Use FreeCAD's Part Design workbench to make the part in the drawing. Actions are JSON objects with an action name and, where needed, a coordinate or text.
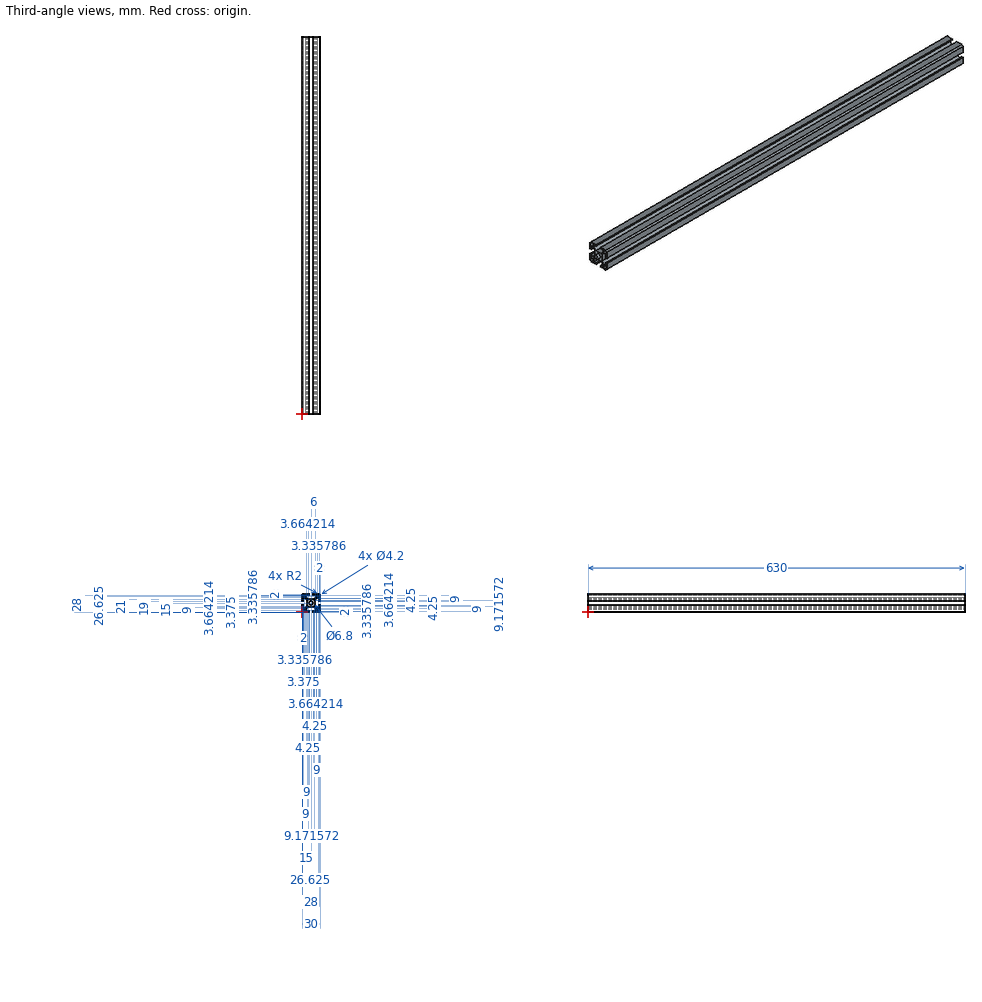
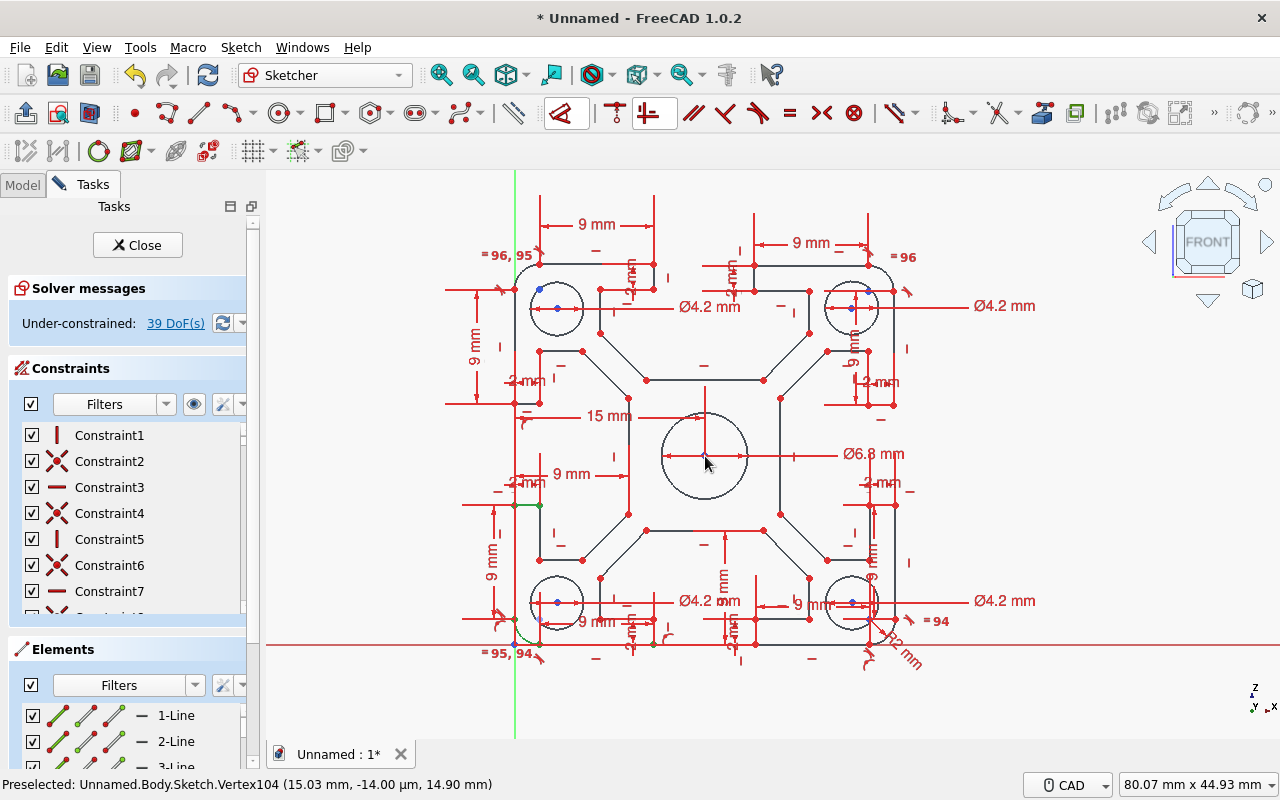
{"action": "left_click", "coordinate": [705, 456]}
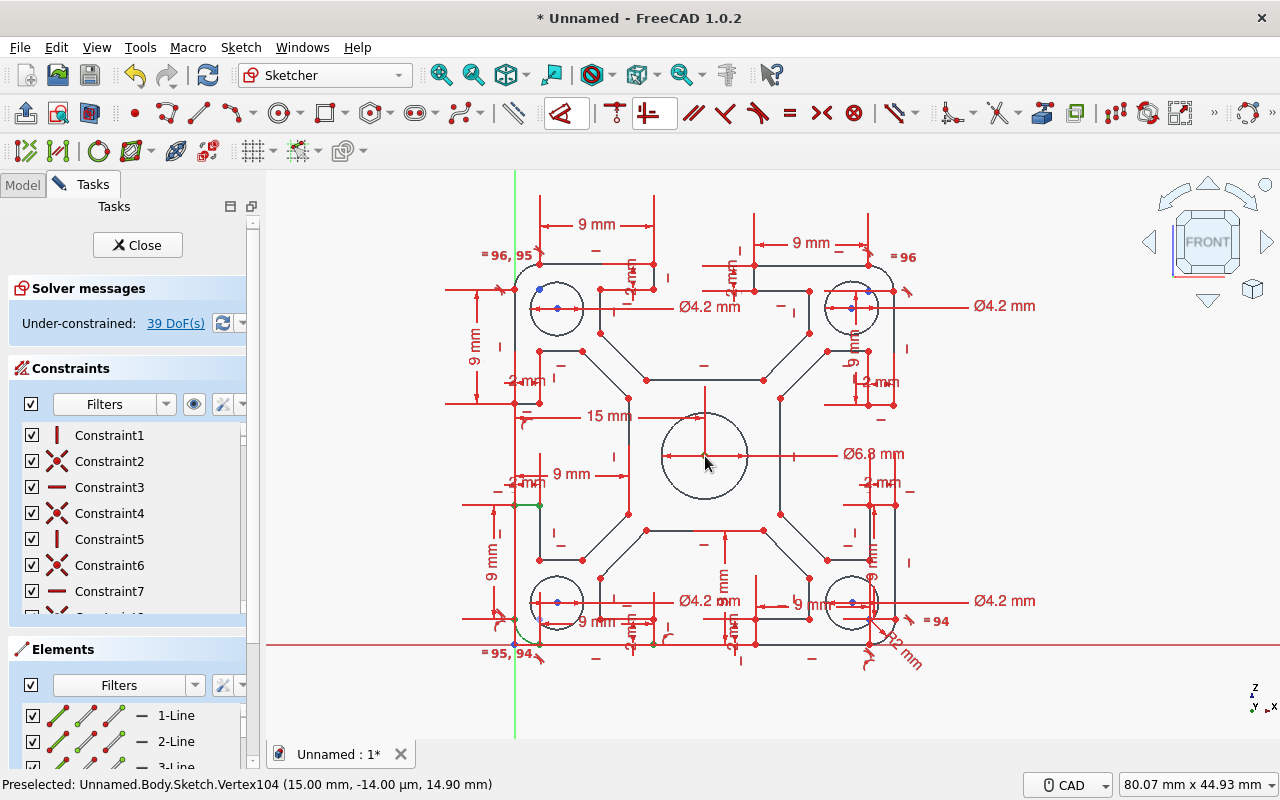
{"action": "left_click", "coordinate": [584, 114]}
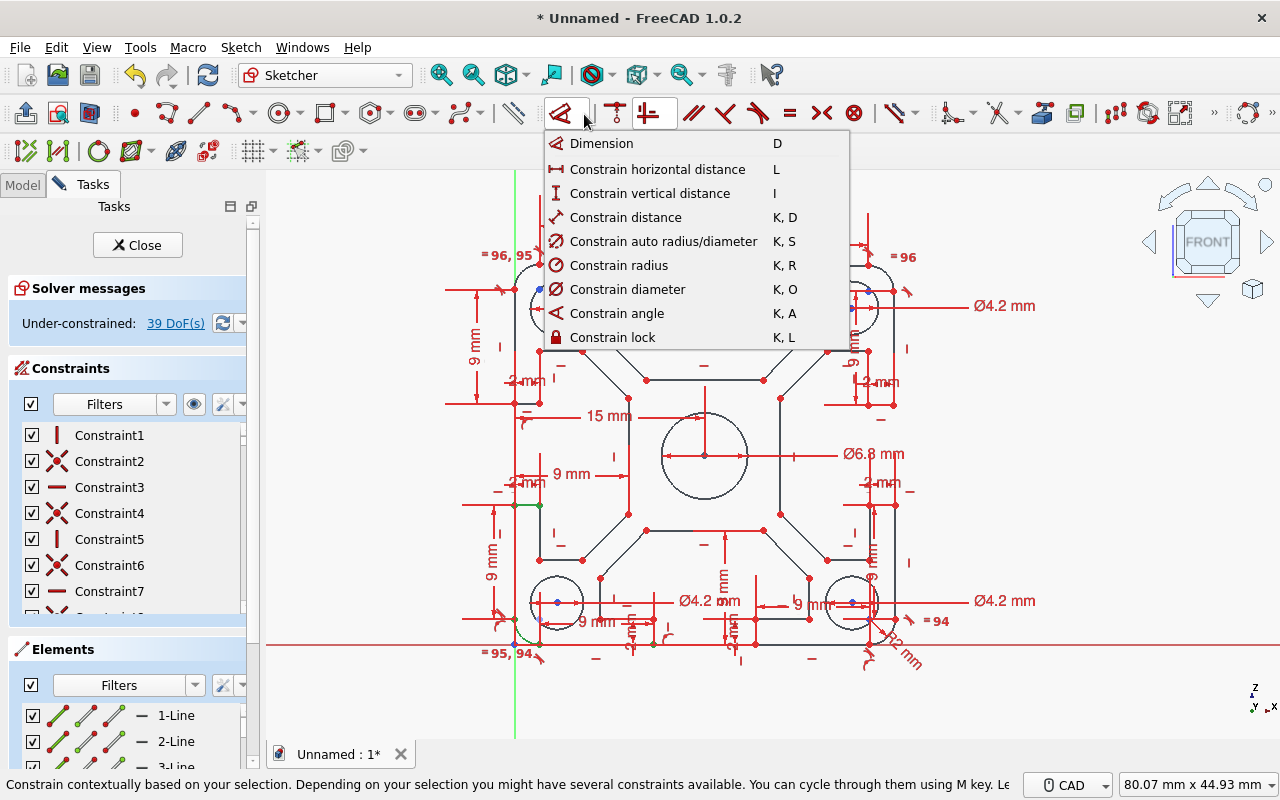
{"action": "left_click", "coordinate": [697, 193]}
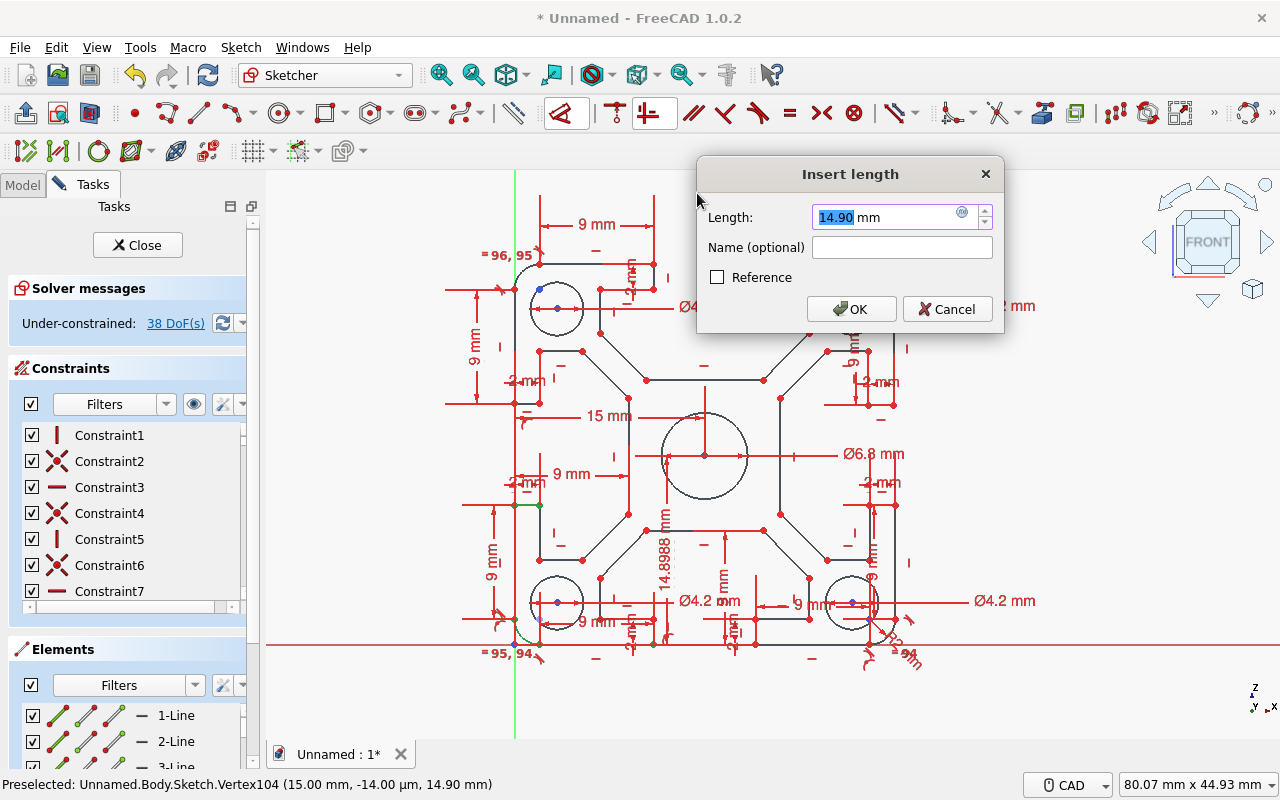
{"action": "type", "text": "15"}
{"action": "key", "text": "Return"}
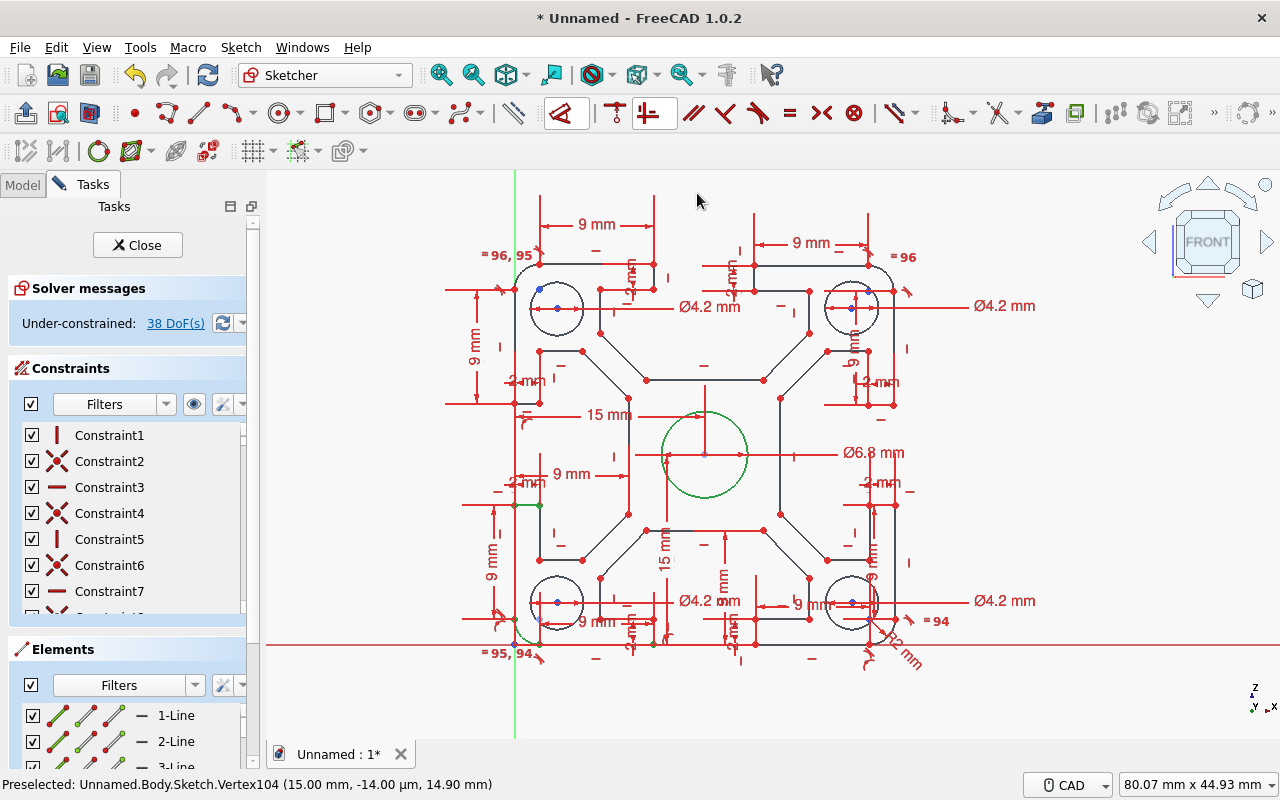
{"action": "left_click", "coordinate": [780, 398]}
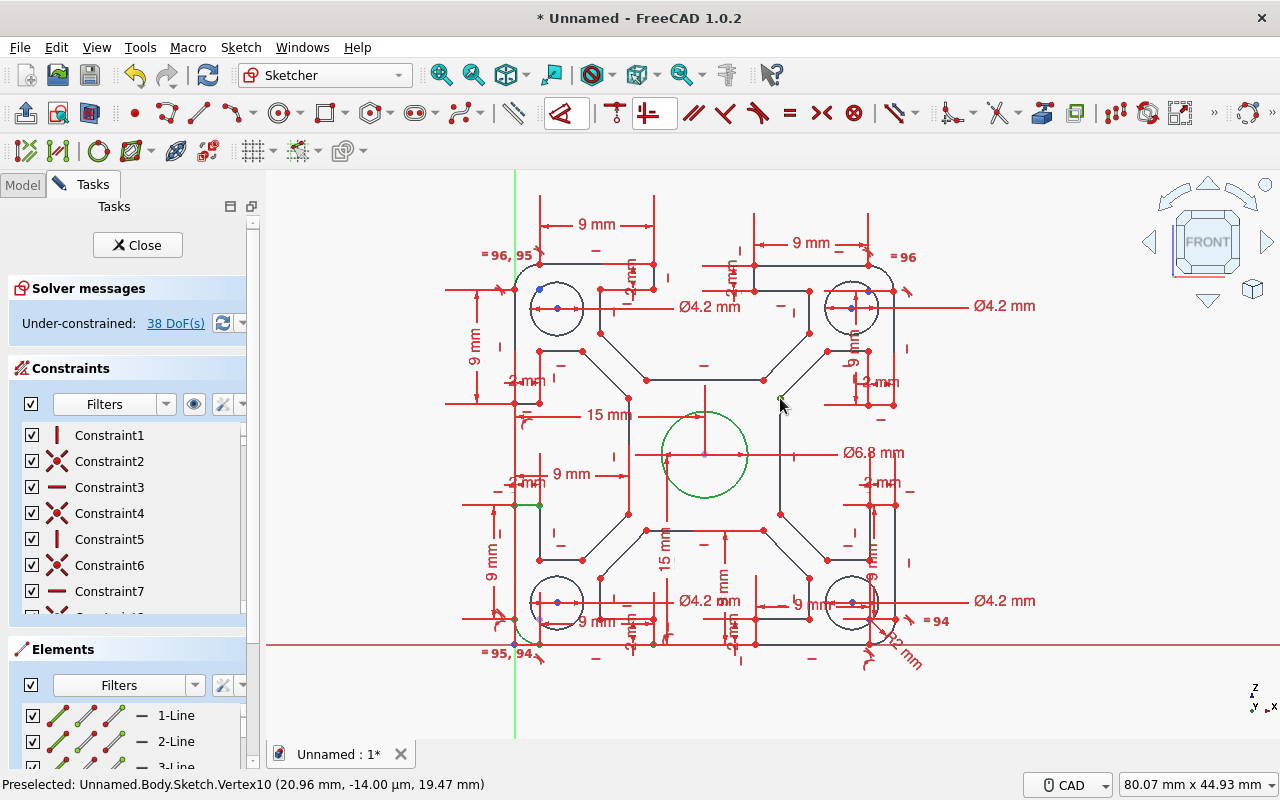
{"action": "left_click", "coordinate": [705, 455]}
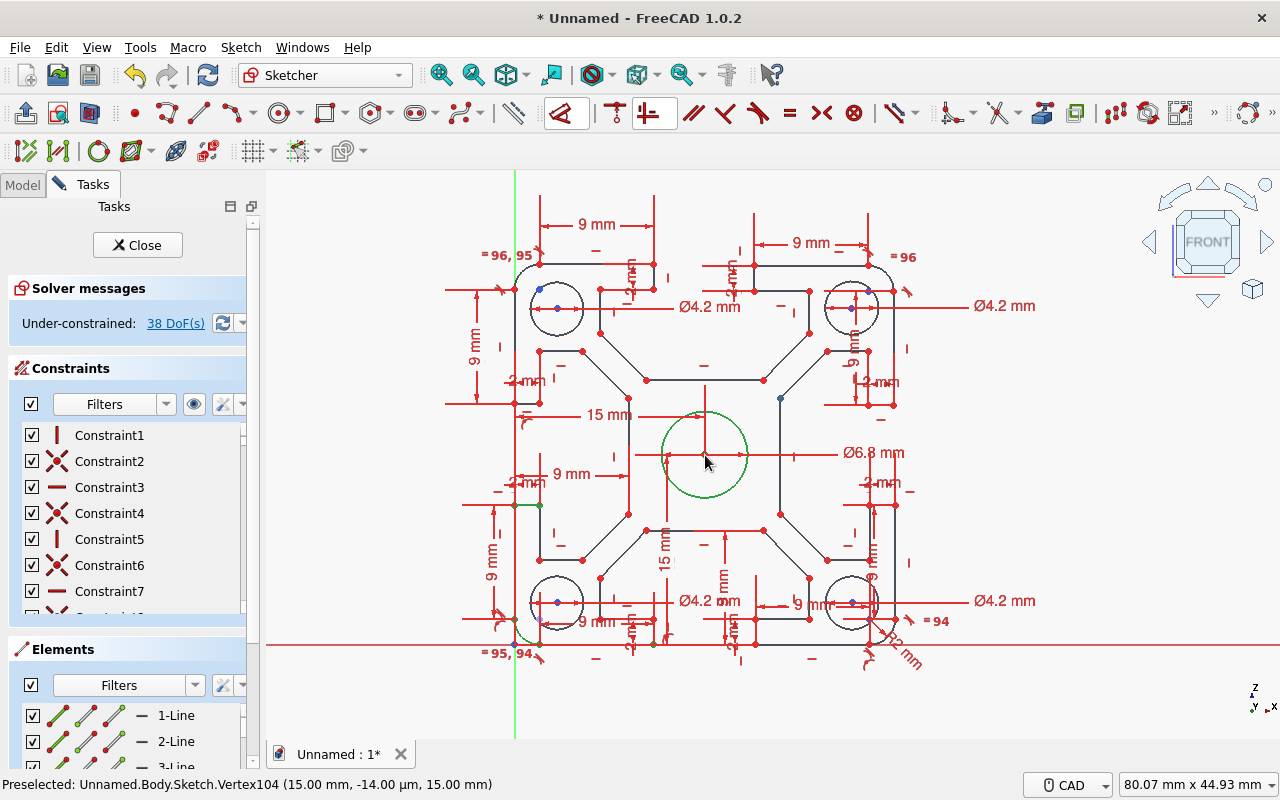
{"action": "left_click", "coordinate": [584, 114]}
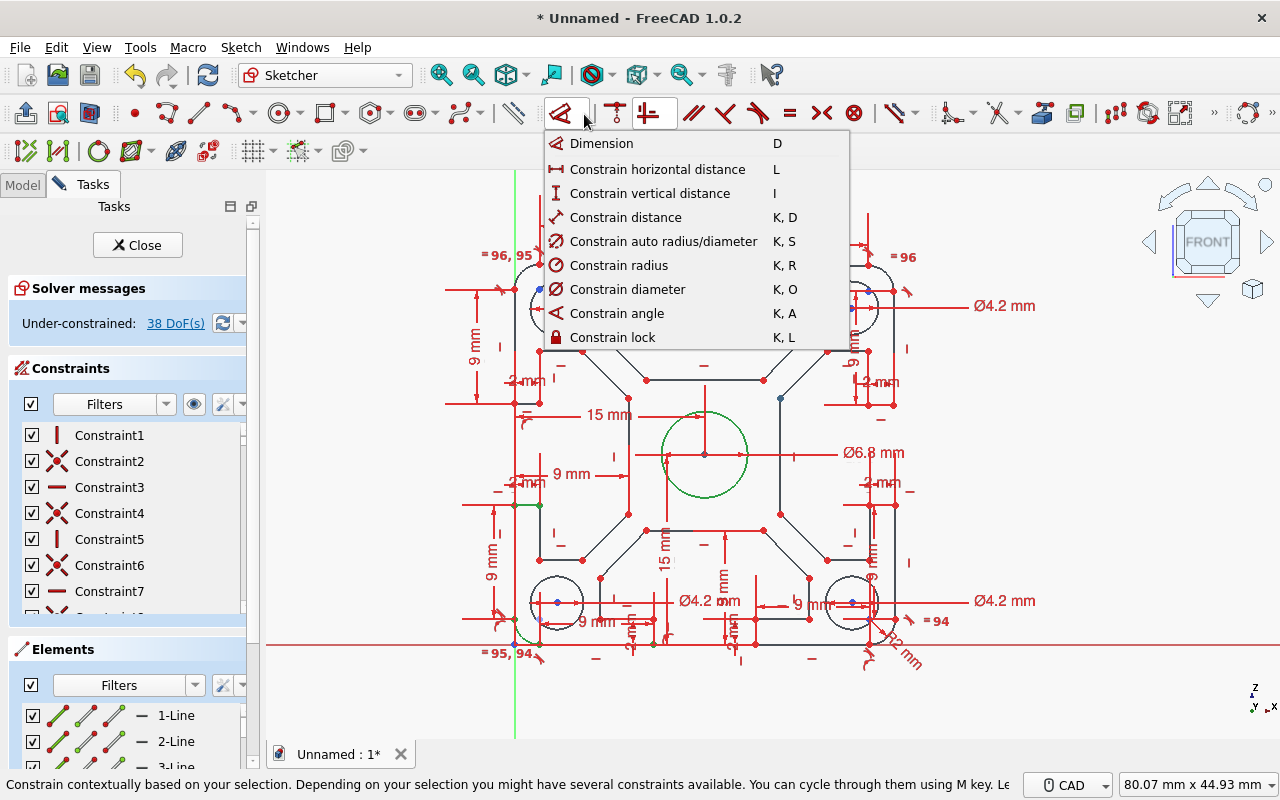
{"action": "left_click", "coordinate": [697, 169]}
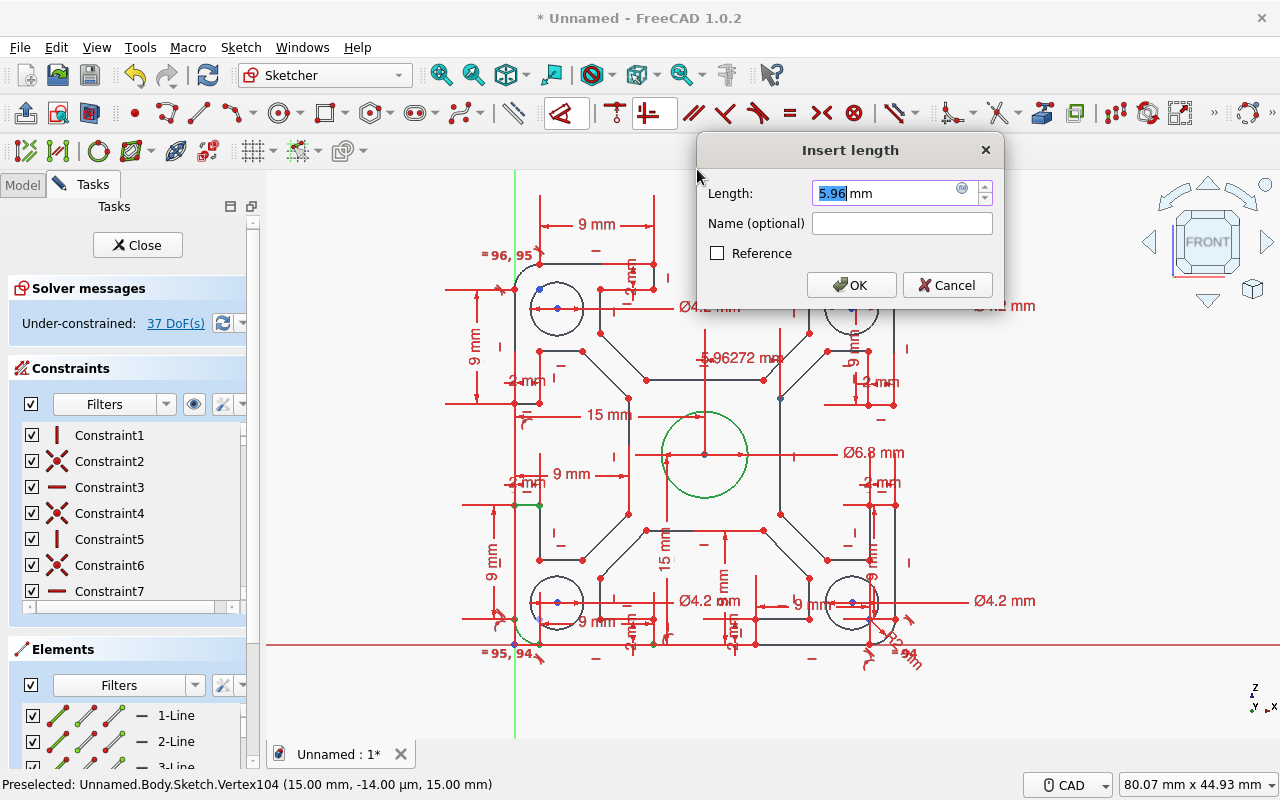
{"action": "type", "text": "6"}
{"action": "key", "text": "Return"}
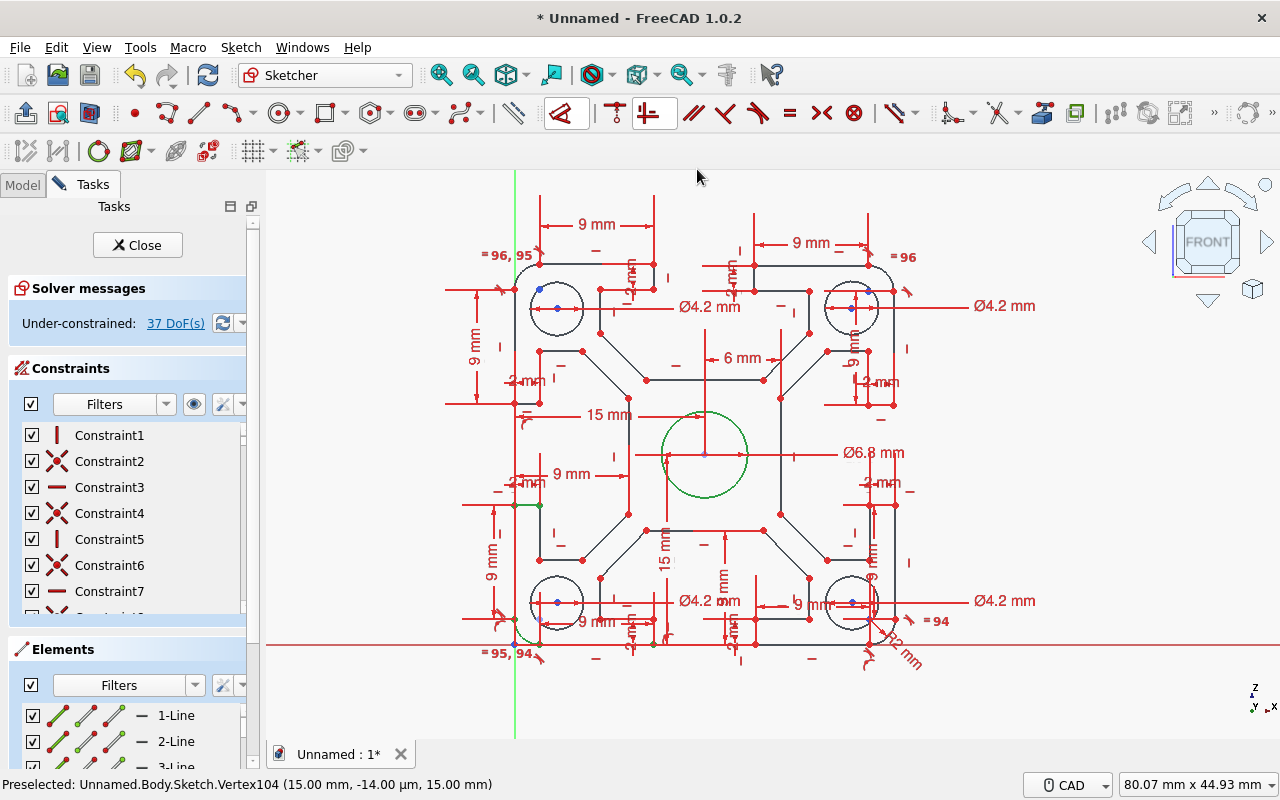
{"action": "left_click", "coordinate": [894, 291]}